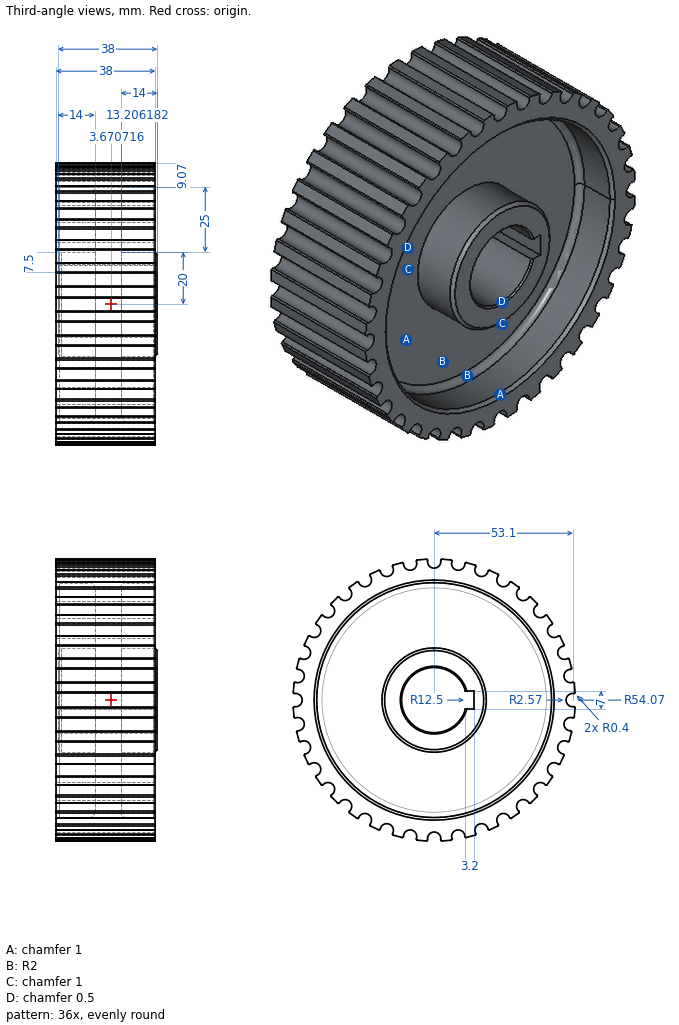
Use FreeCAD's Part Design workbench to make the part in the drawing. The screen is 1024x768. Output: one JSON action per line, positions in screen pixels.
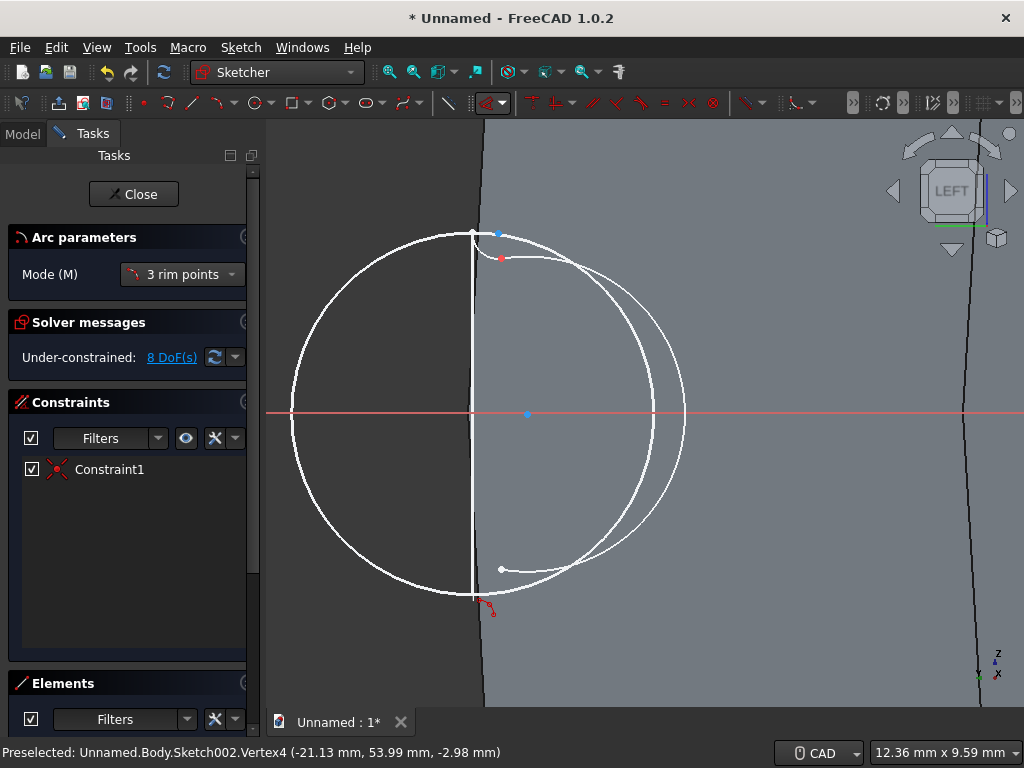
{"action": "scroll", "coordinate": [468, 377], "scroll_direction": "up", "scroll_amount": 7}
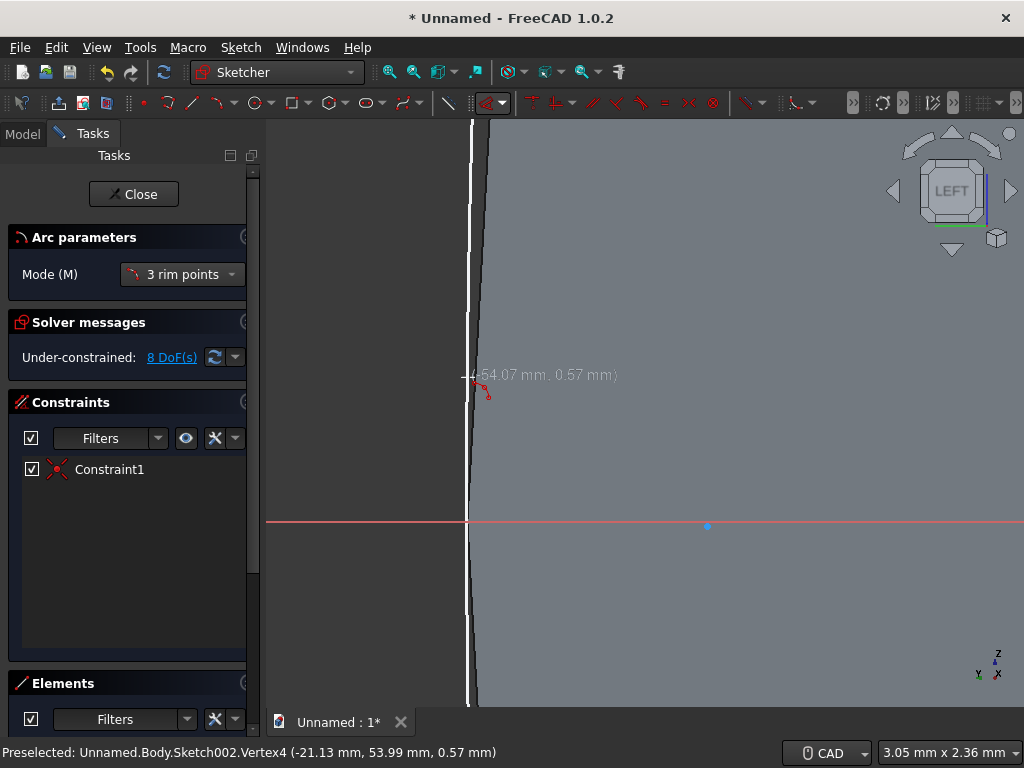
{"action": "left_click", "coordinate": [468, 375]}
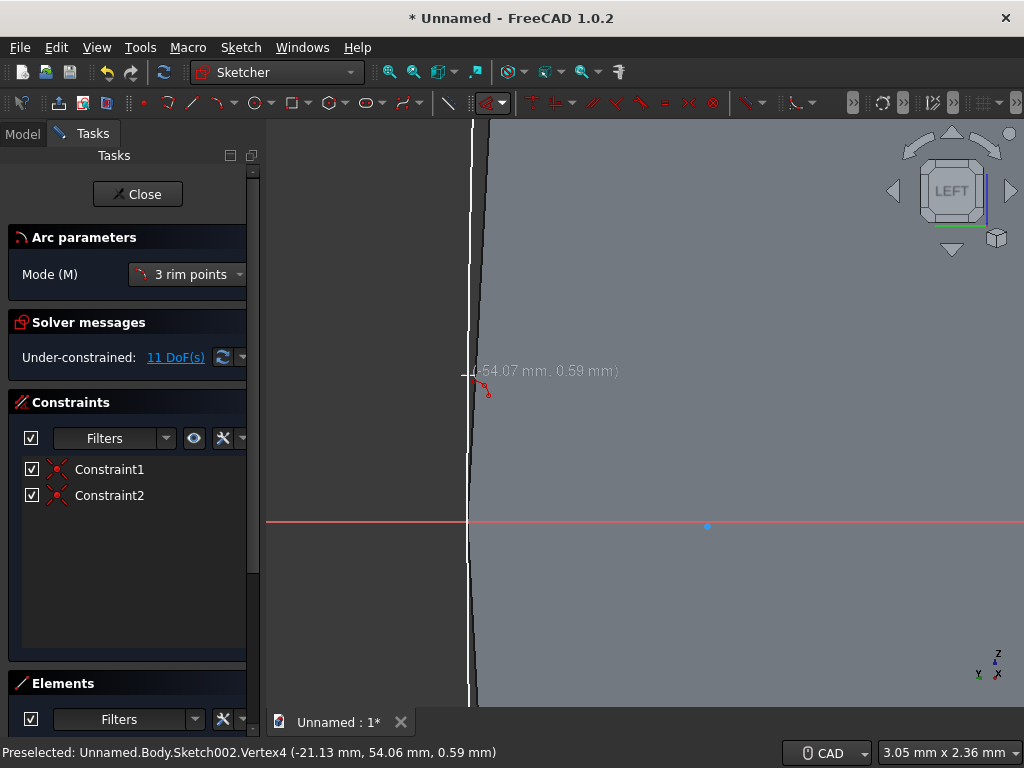
{"action": "scroll", "coordinate": [468, 377], "scroll_direction": "down", "scroll_amount": 7}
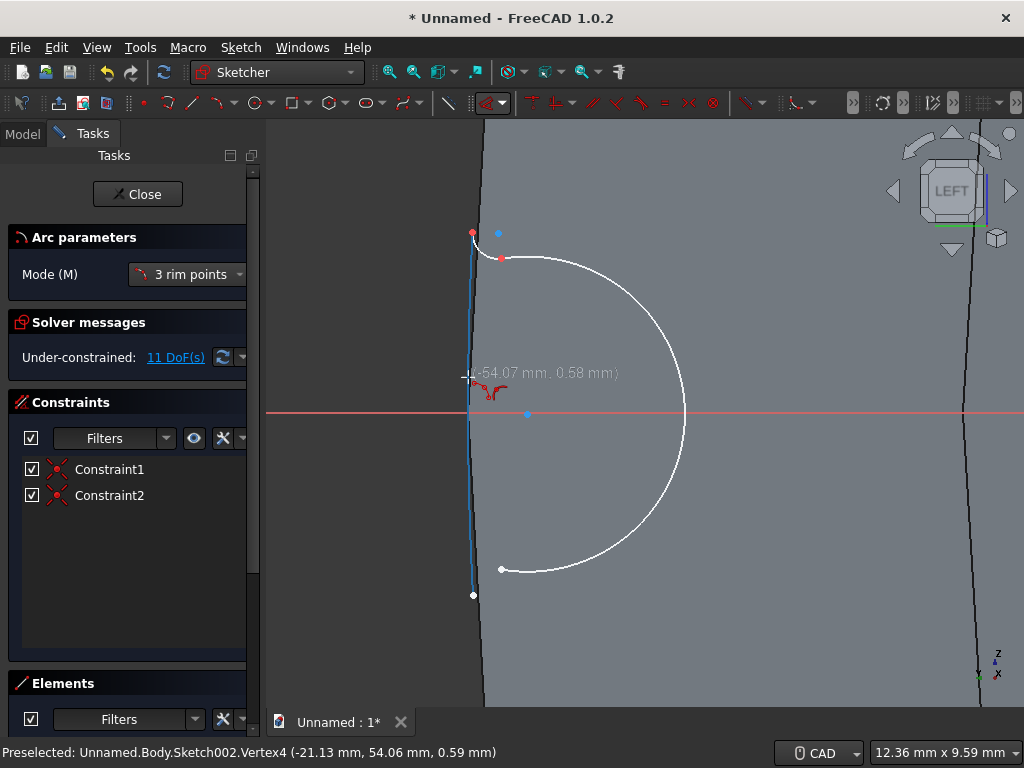
{"action": "left_click", "coordinate": [473, 595]}
{"action": "left_click", "coordinate": [502, 570]}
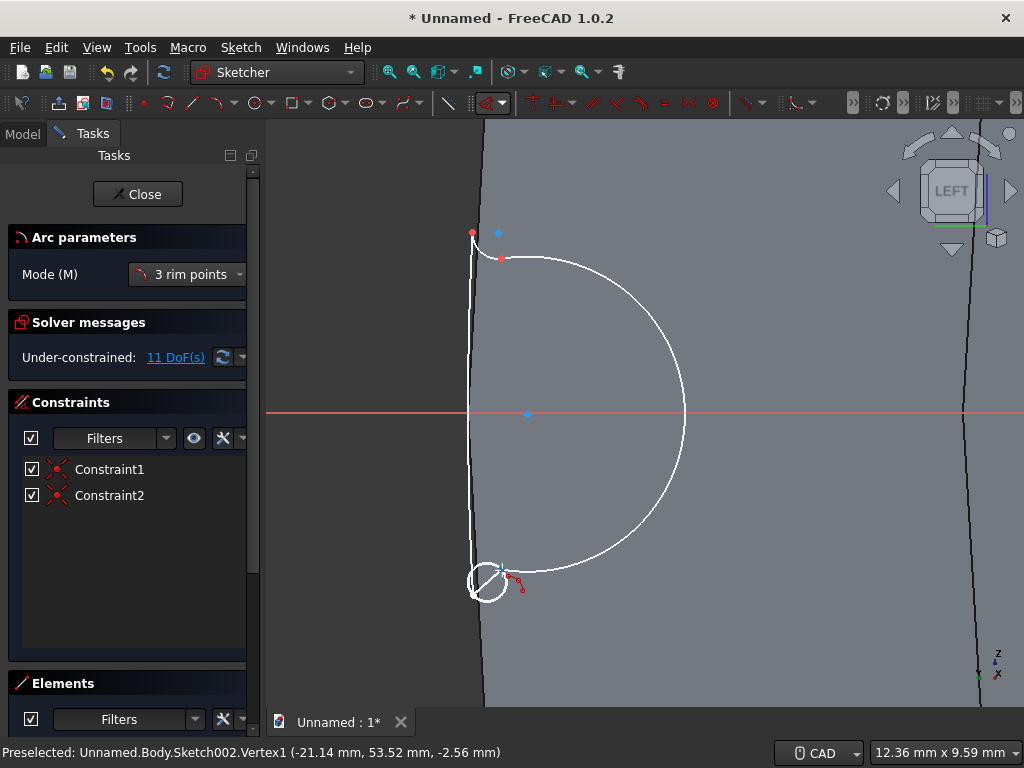
{"action": "scroll", "coordinate": [481, 574], "scroll_direction": "up", "scroll_amount": 3}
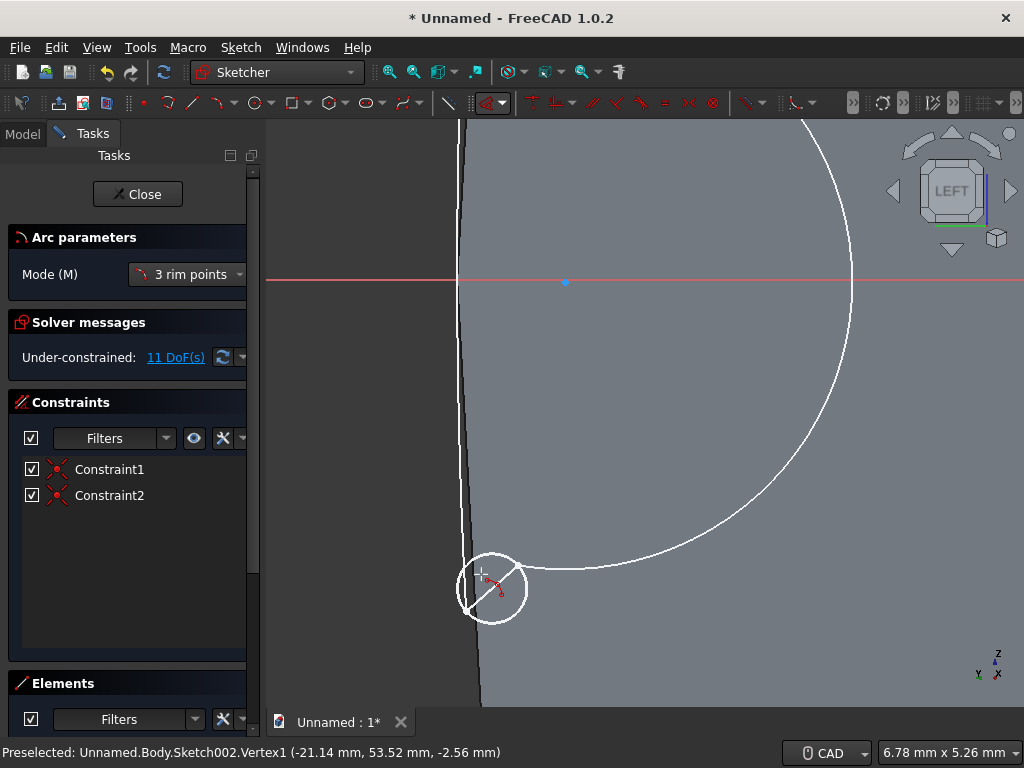
{"action": "left_click", "coordinate": [481, 574]}
{"action": "key", "text": "Escape"}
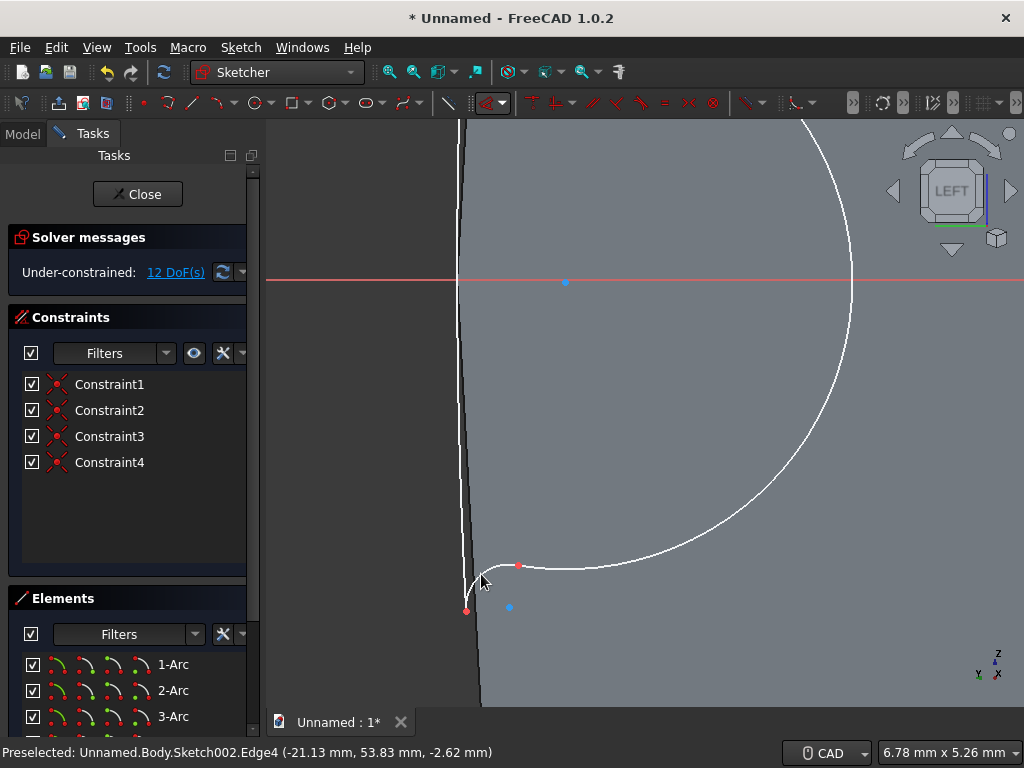
{"action": "left_click", "coordinate": [786, 466]}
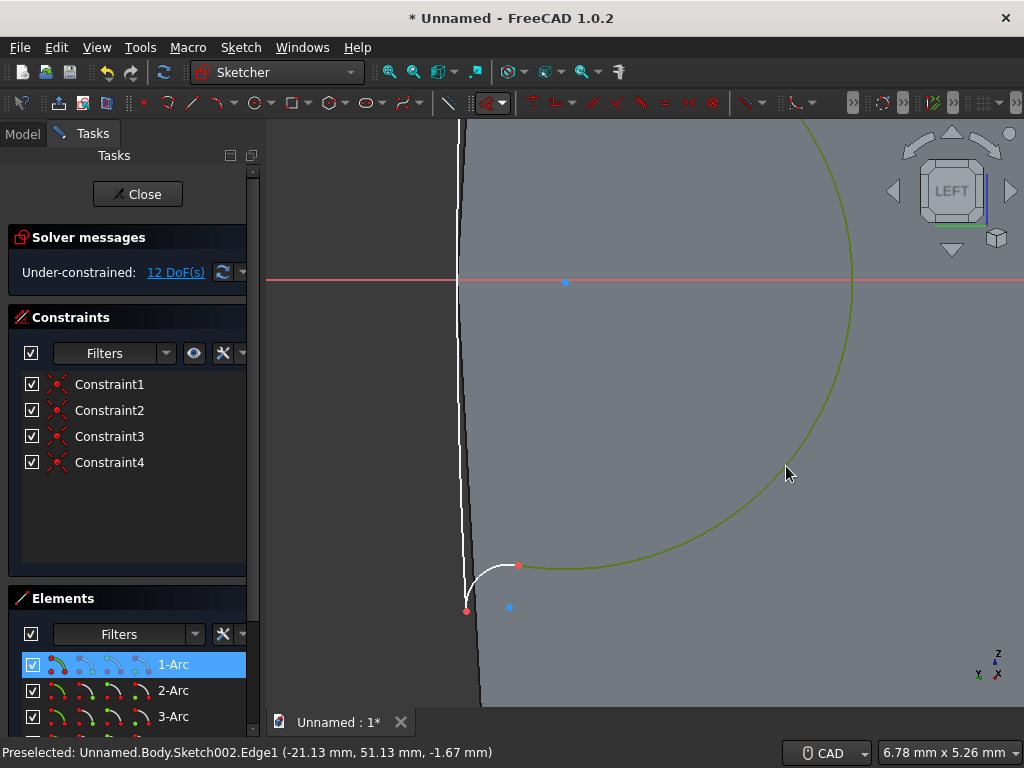
{"action": "scroll", "coordinate": [481, 575], "scroll_direction": "down", "scroll_amount": 3}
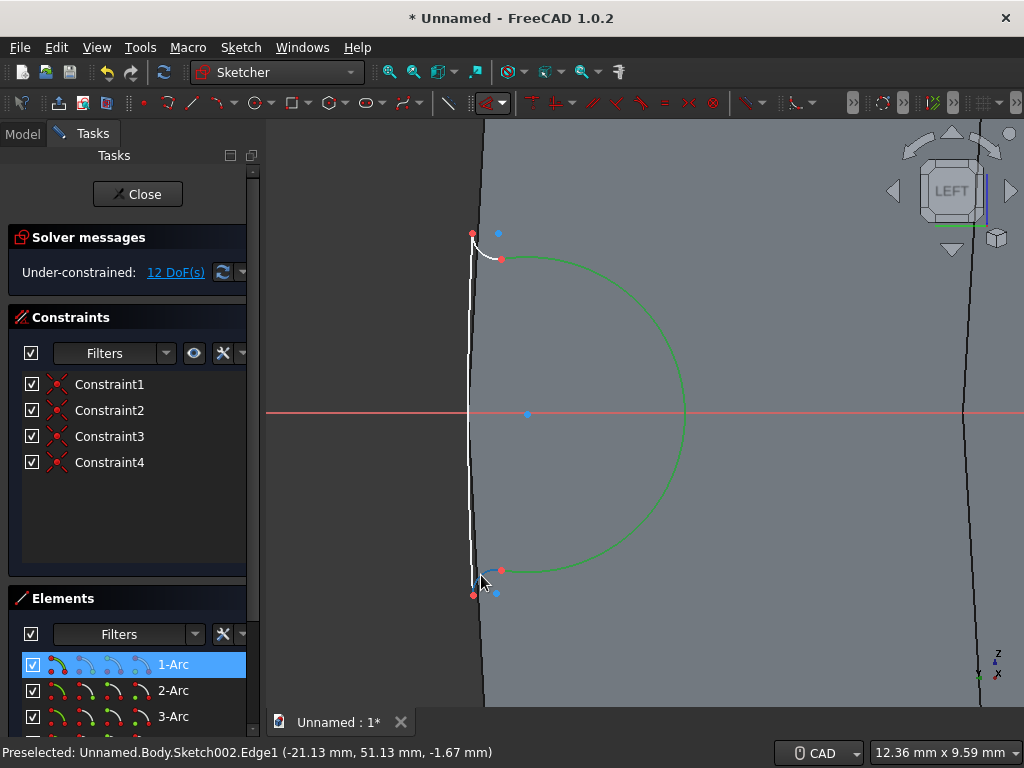
{"action": "left_click", "coordinate": [489, 257]}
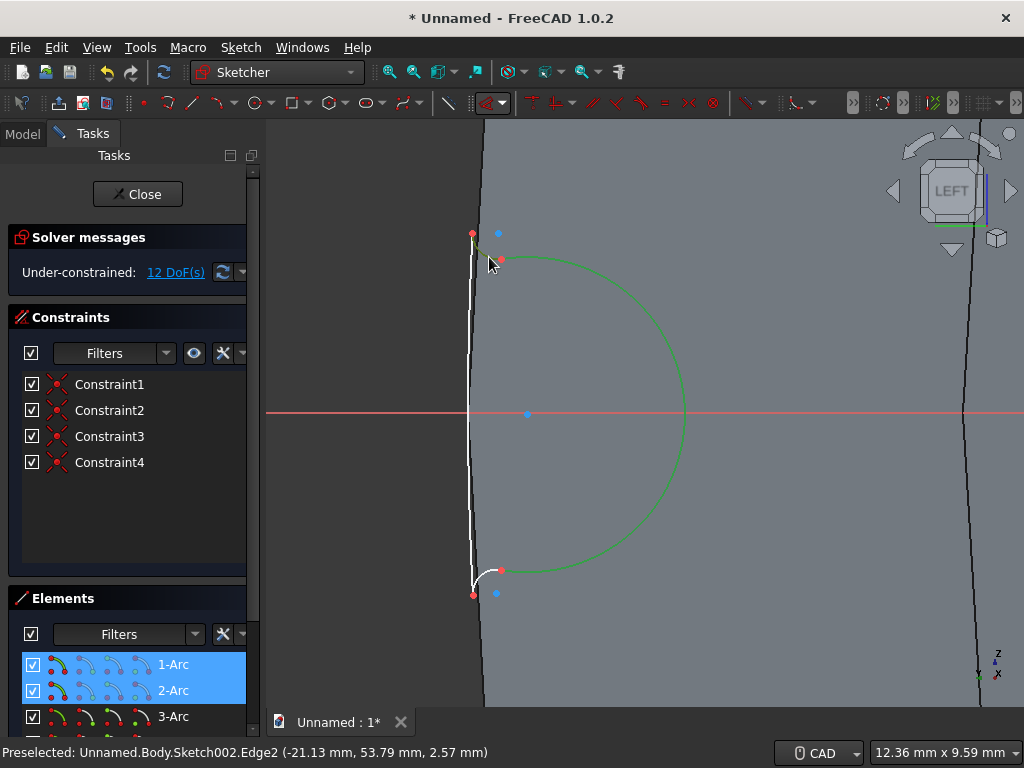
{"action": "left_click", "coordinate": [642, 104]}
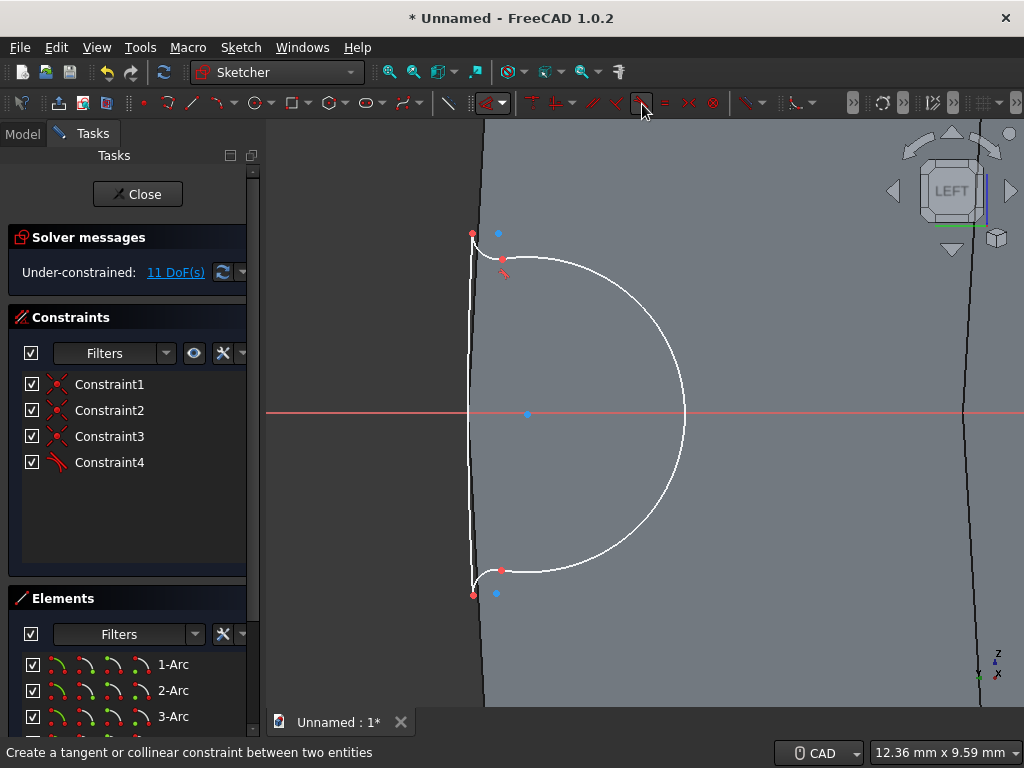
{"action": "left_click", "coordinate": [648, 516]}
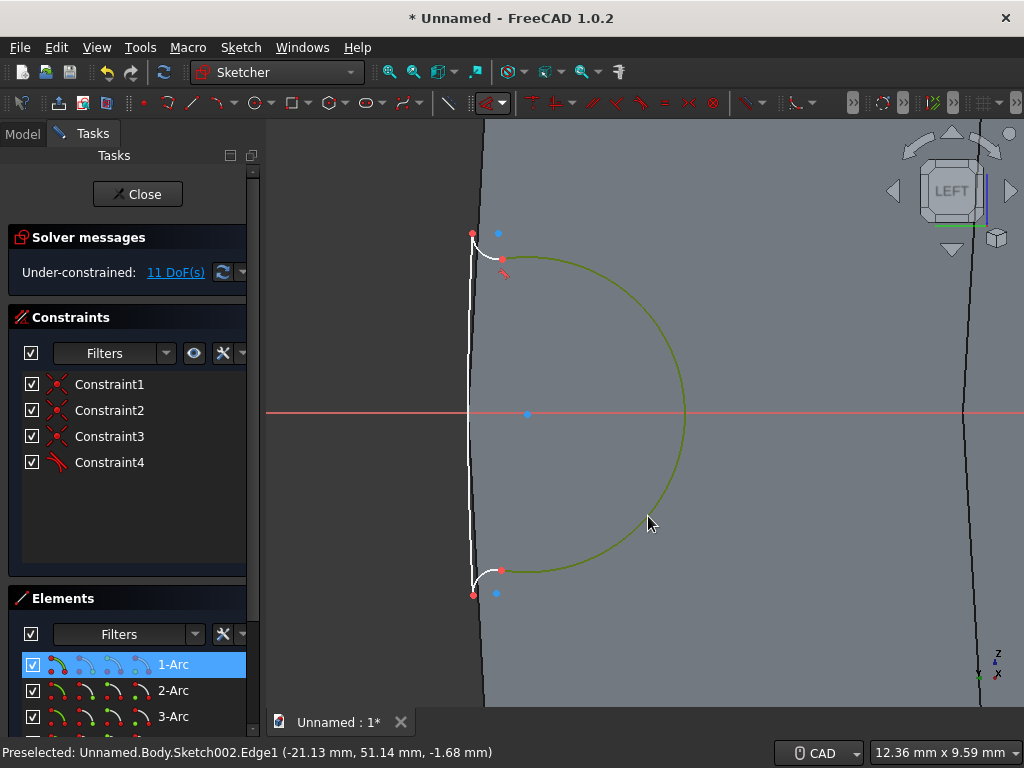
{"action": "left_click", "coordinate": [488, 571]}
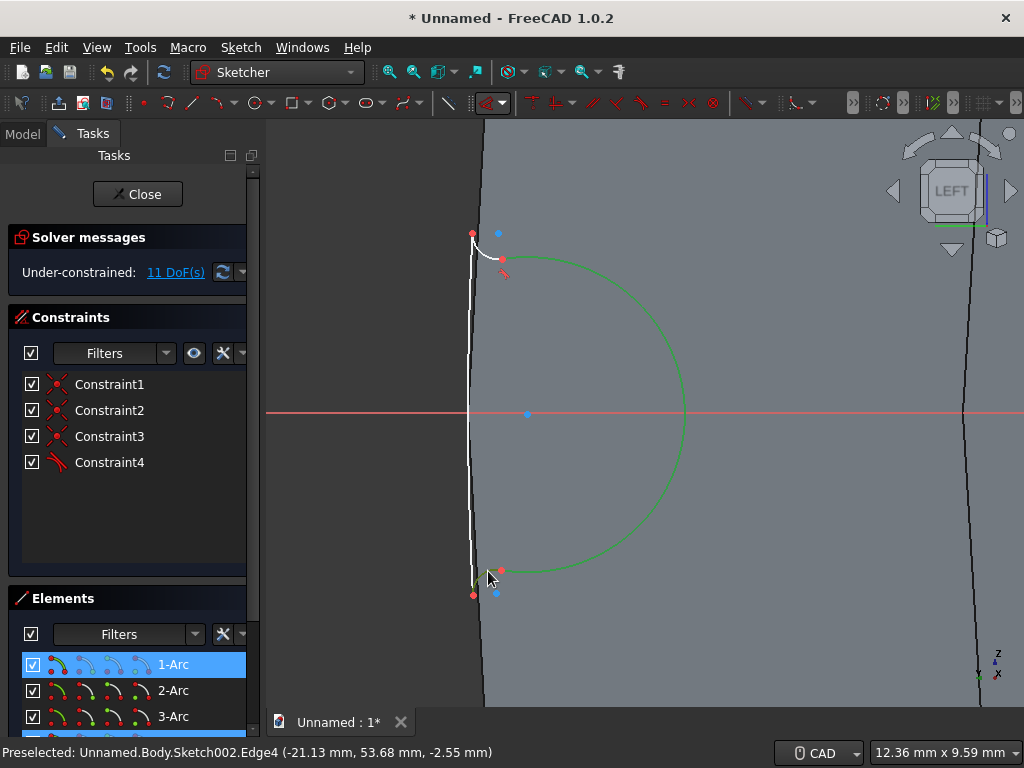
{"action": "left_click", "coordinate": [642, 104]}